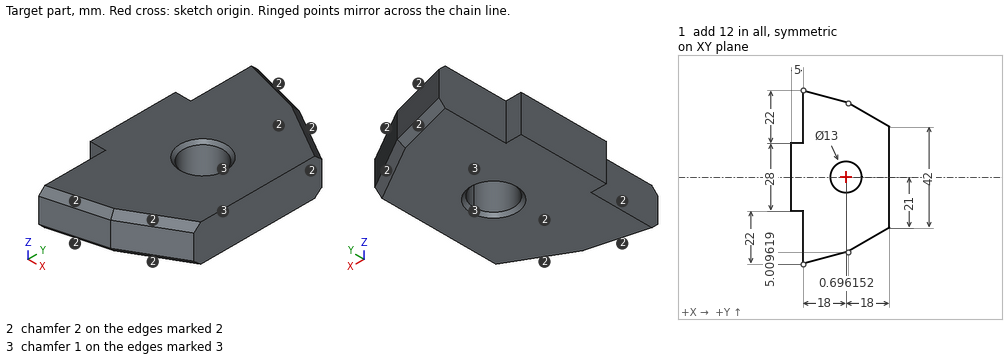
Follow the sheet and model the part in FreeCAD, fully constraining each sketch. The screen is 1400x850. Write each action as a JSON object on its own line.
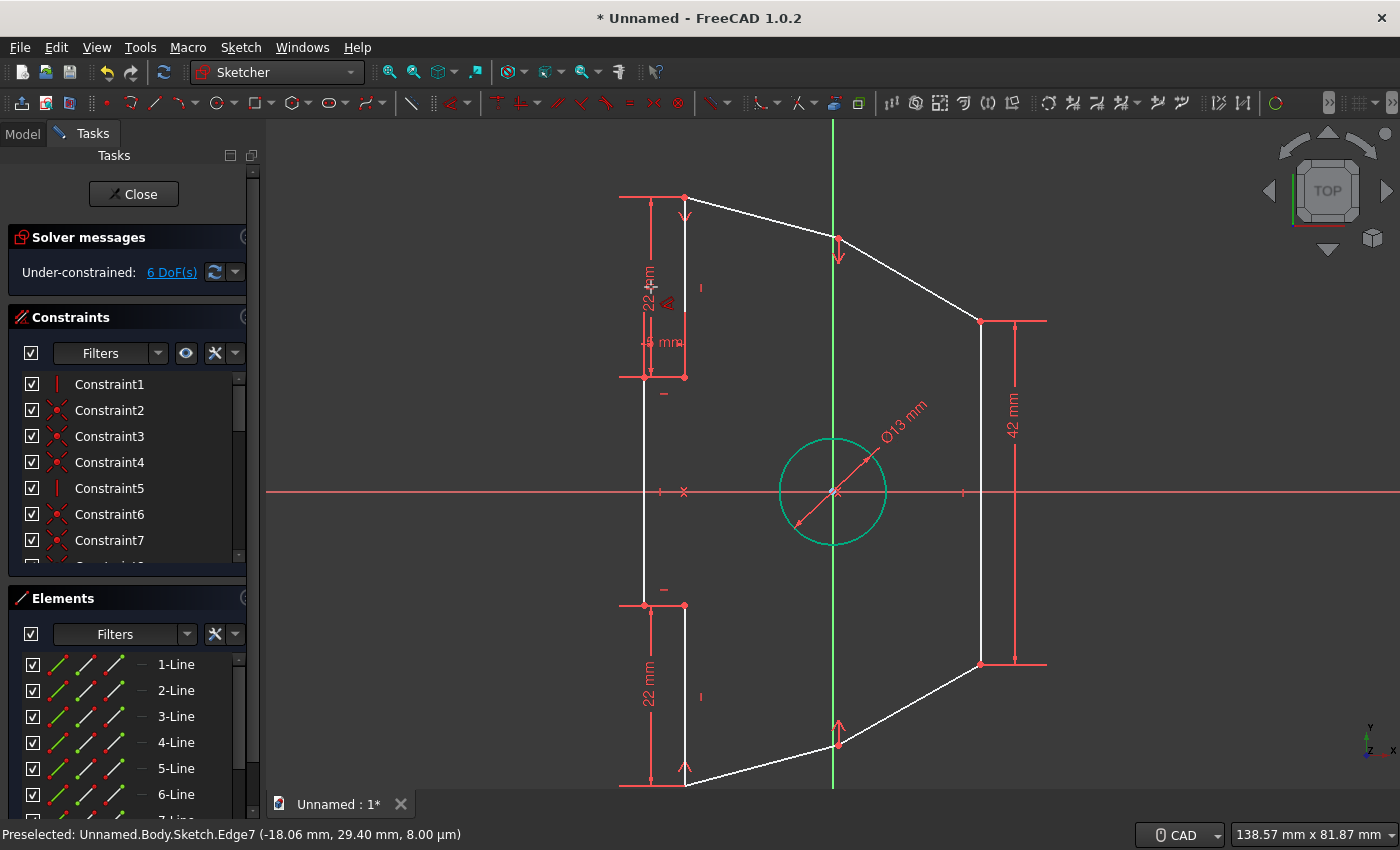
{"action": "left_click", "coordinate": [644, 446]}
{"action": "left_click", "coordinate": [610, 439]}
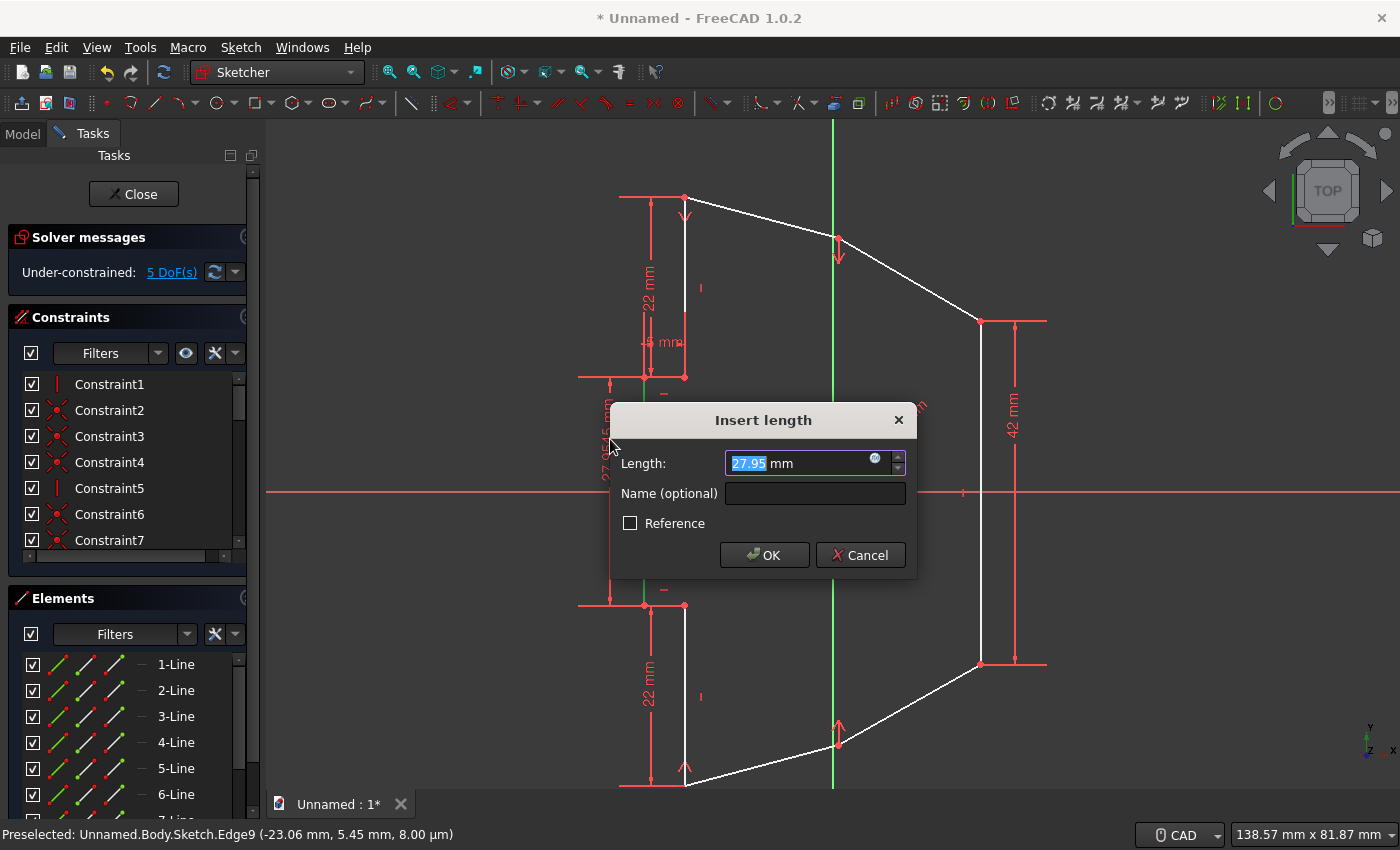
{"action": "type", "text": "28"}
{"action": "key", "text": "Return"}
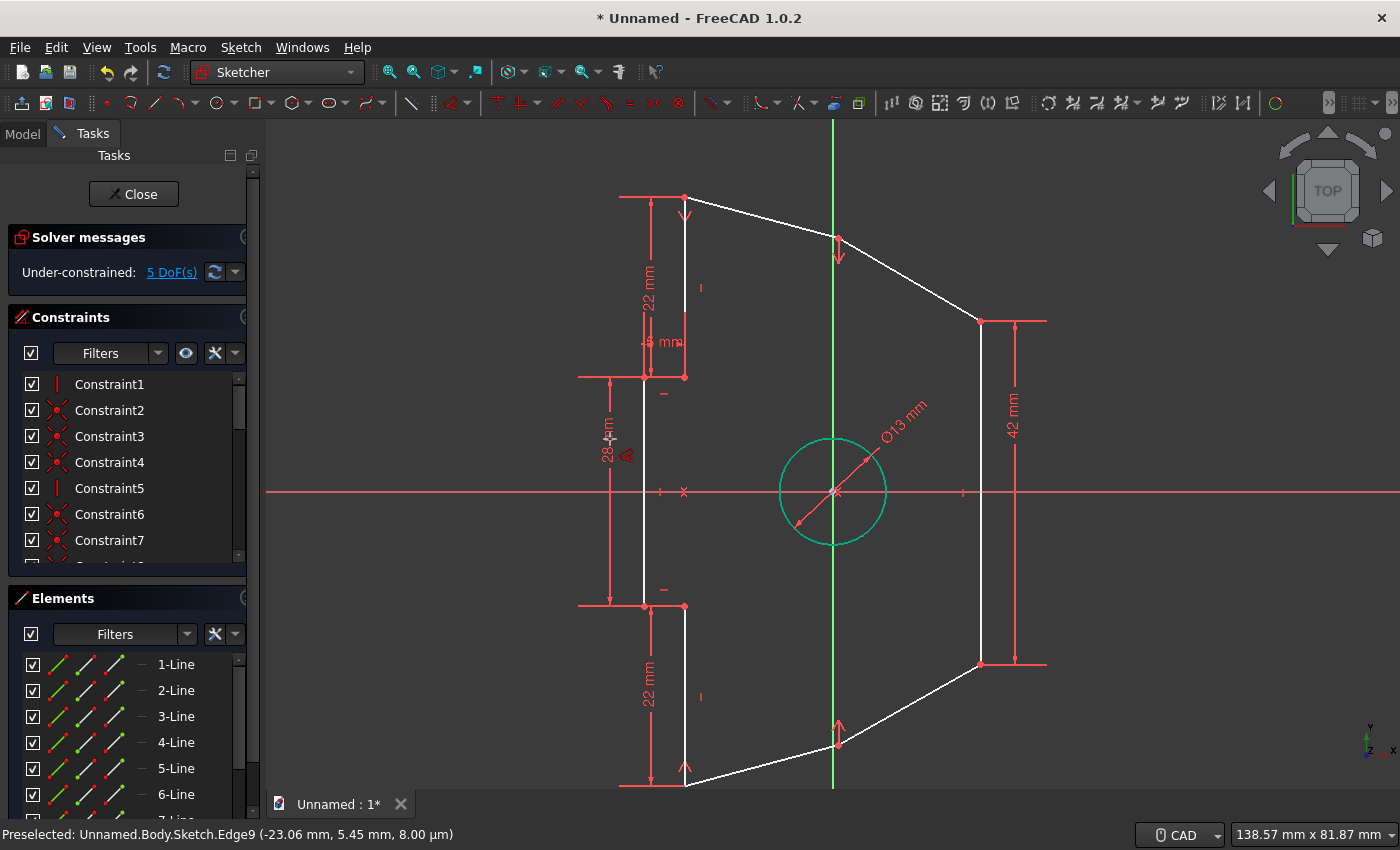
{"action": "left_click", "coordinate": [685, 606]}
{"action": "left_click", "coordinate": [759, 640]}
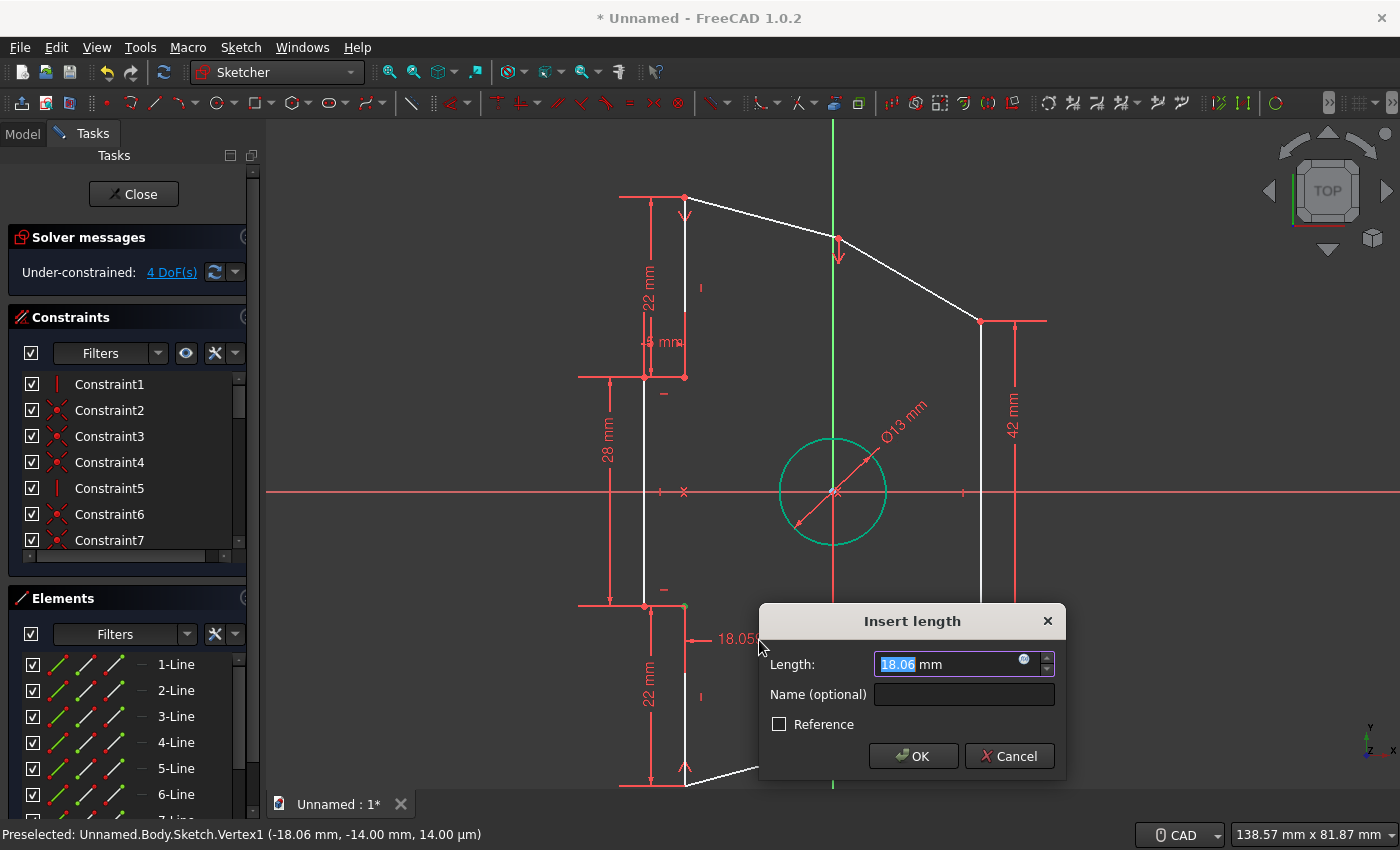
{"action": "type", "text": "18"}
{"action": "key", "text": "Return"}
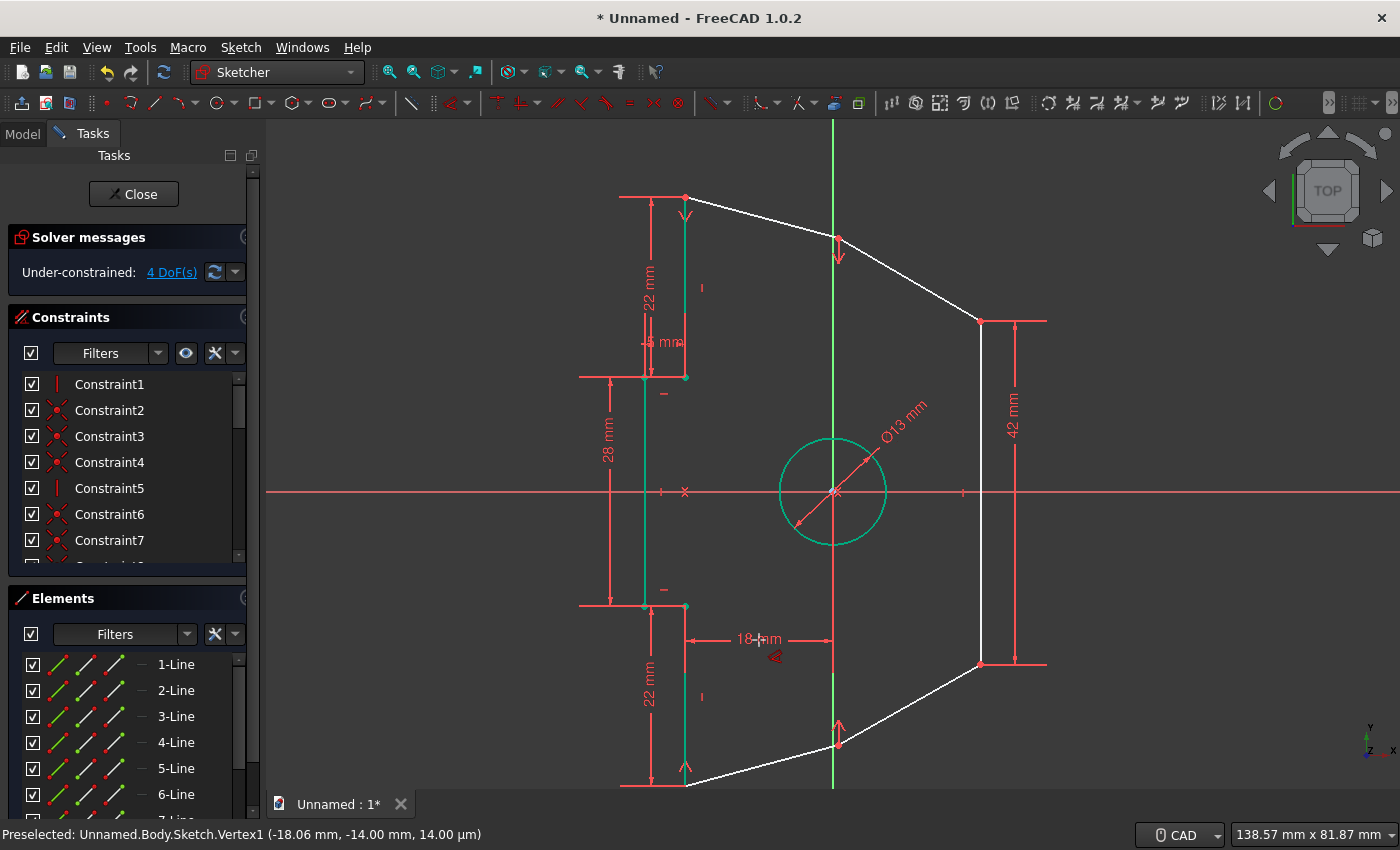
{"action": "left_click", "coordinate": [981, 665]}
{"action": "left_click", "coordinate": [873, 699]}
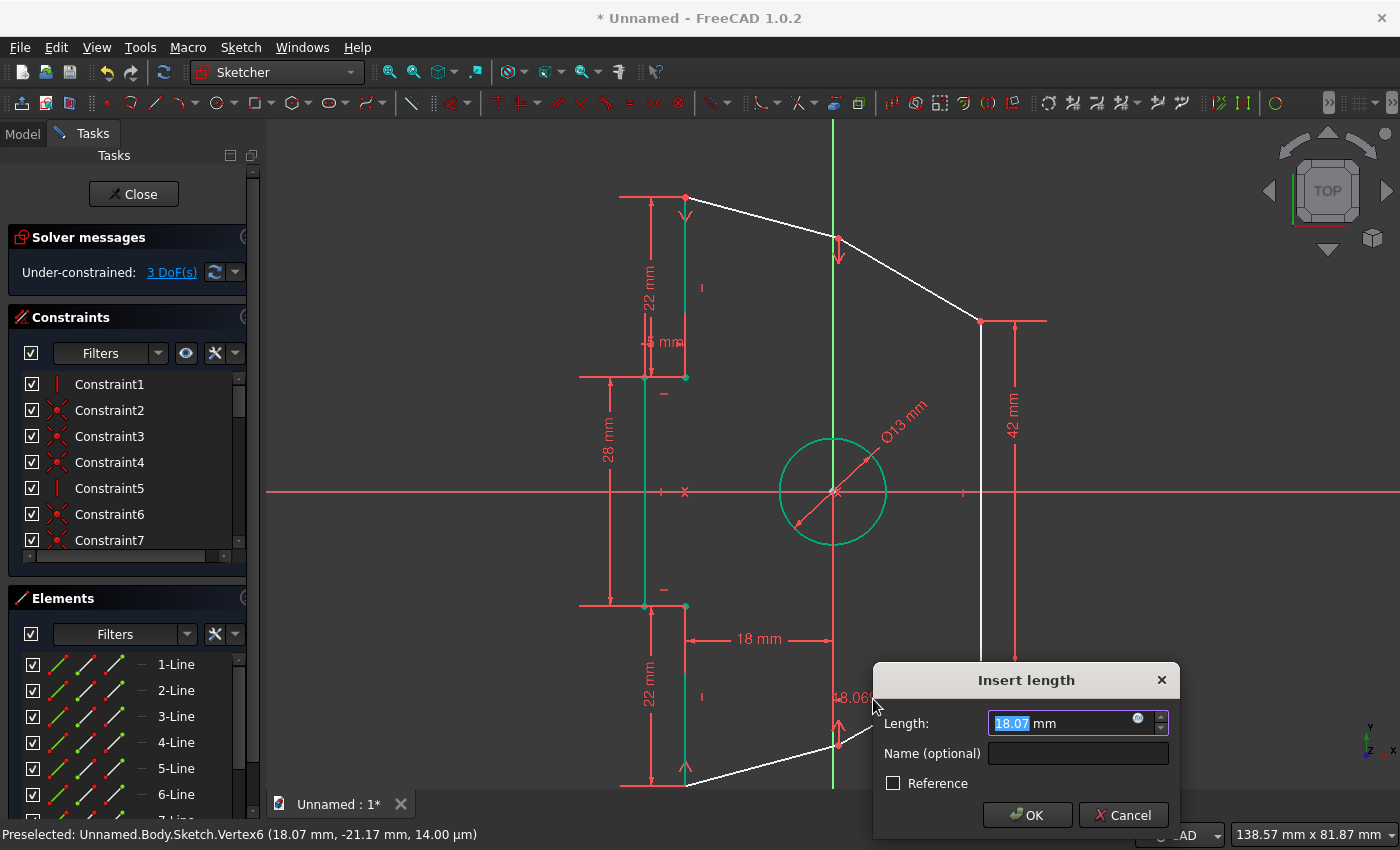
{"action": "type", "text": "18"}
{"action": "key", "text": "Return"}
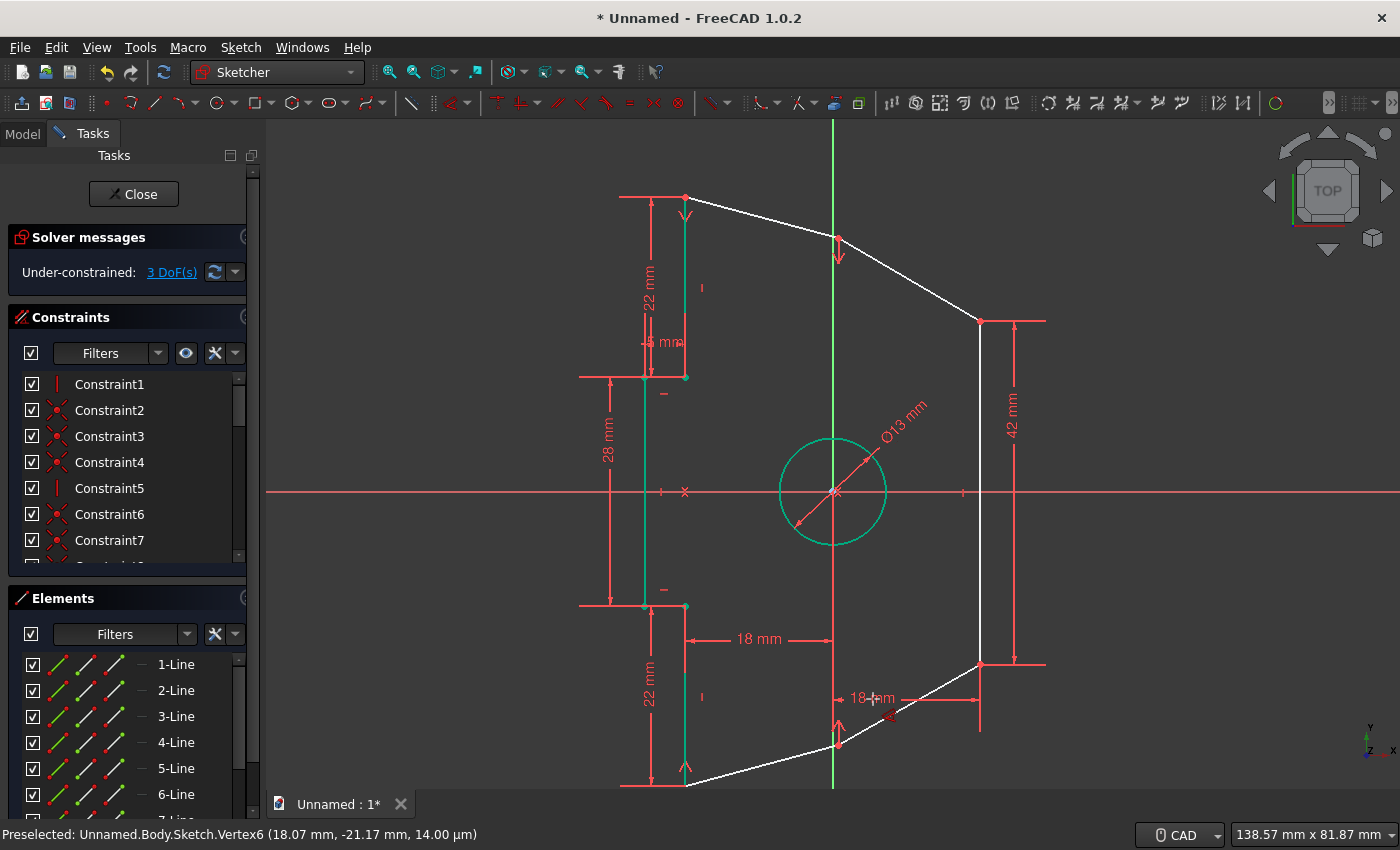
{"action": "left_click", "coordinate": [980, 665]}
{"action": "left_click", "coordinate": [1014, 578]}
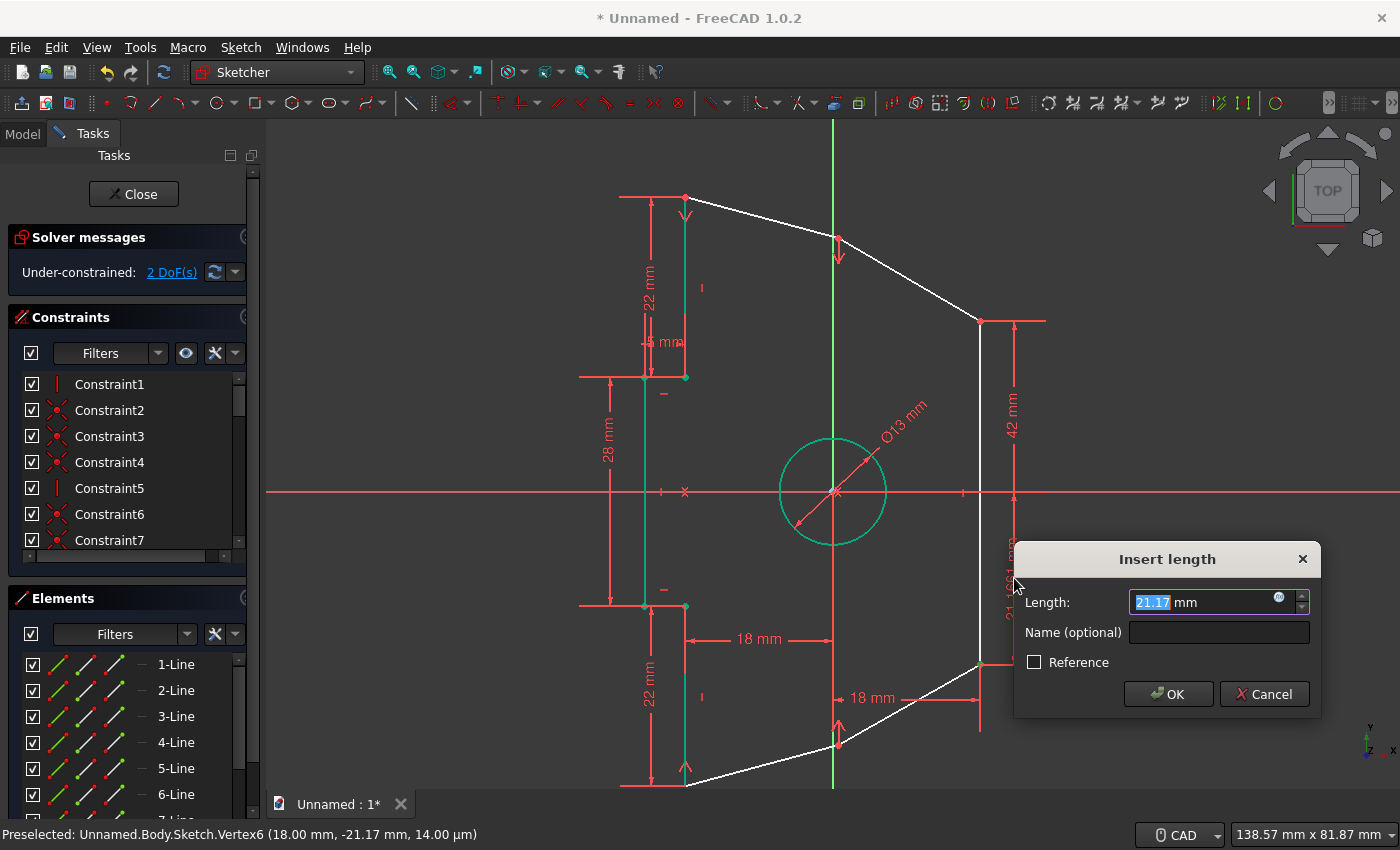
{"action": "type", "text": "21"}
{"action": "key", "text": "Return"}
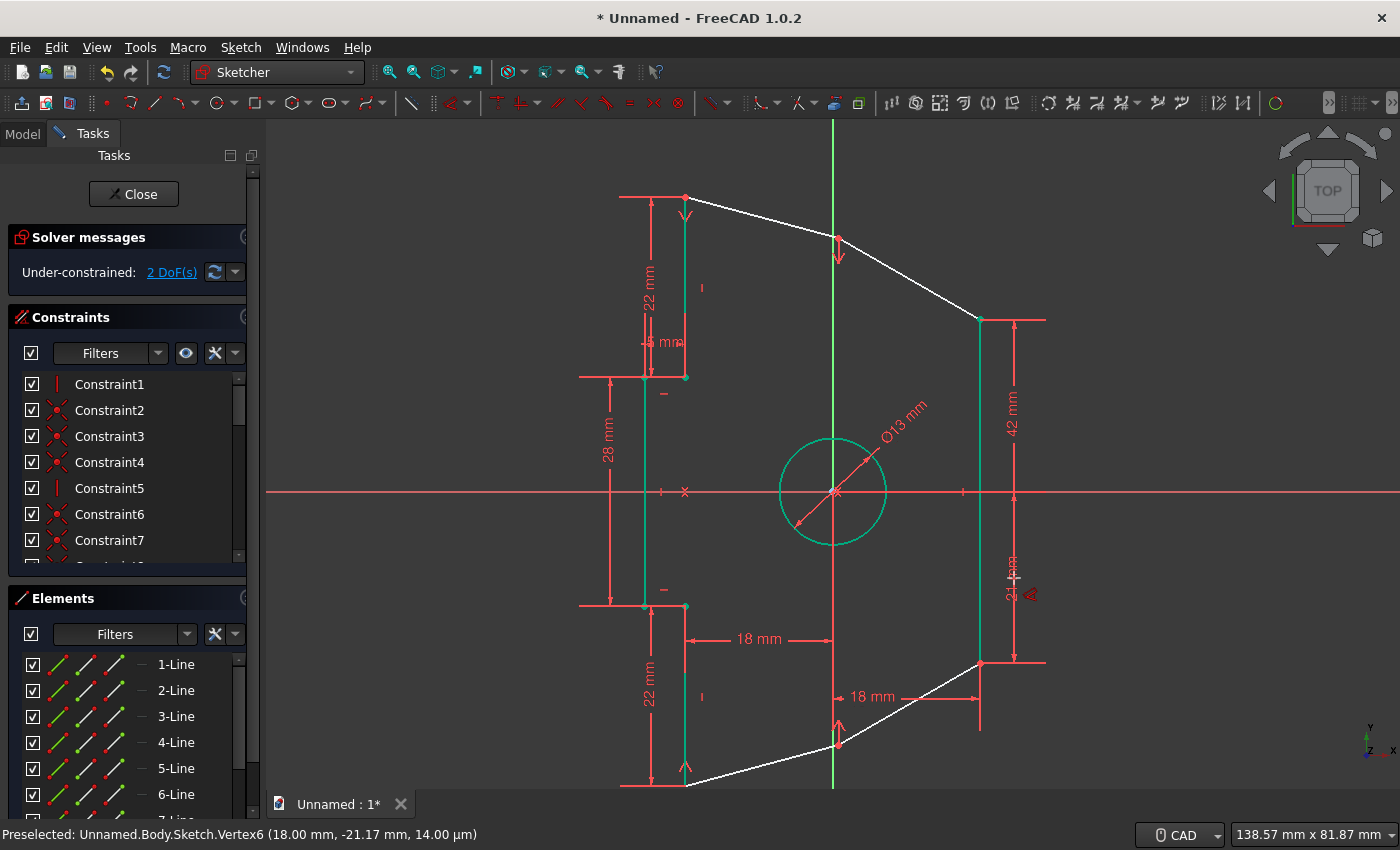
{"action": "scroll", "coordinate": [839, 745], "scroll_direction": "up", "scroll_amount": 10}